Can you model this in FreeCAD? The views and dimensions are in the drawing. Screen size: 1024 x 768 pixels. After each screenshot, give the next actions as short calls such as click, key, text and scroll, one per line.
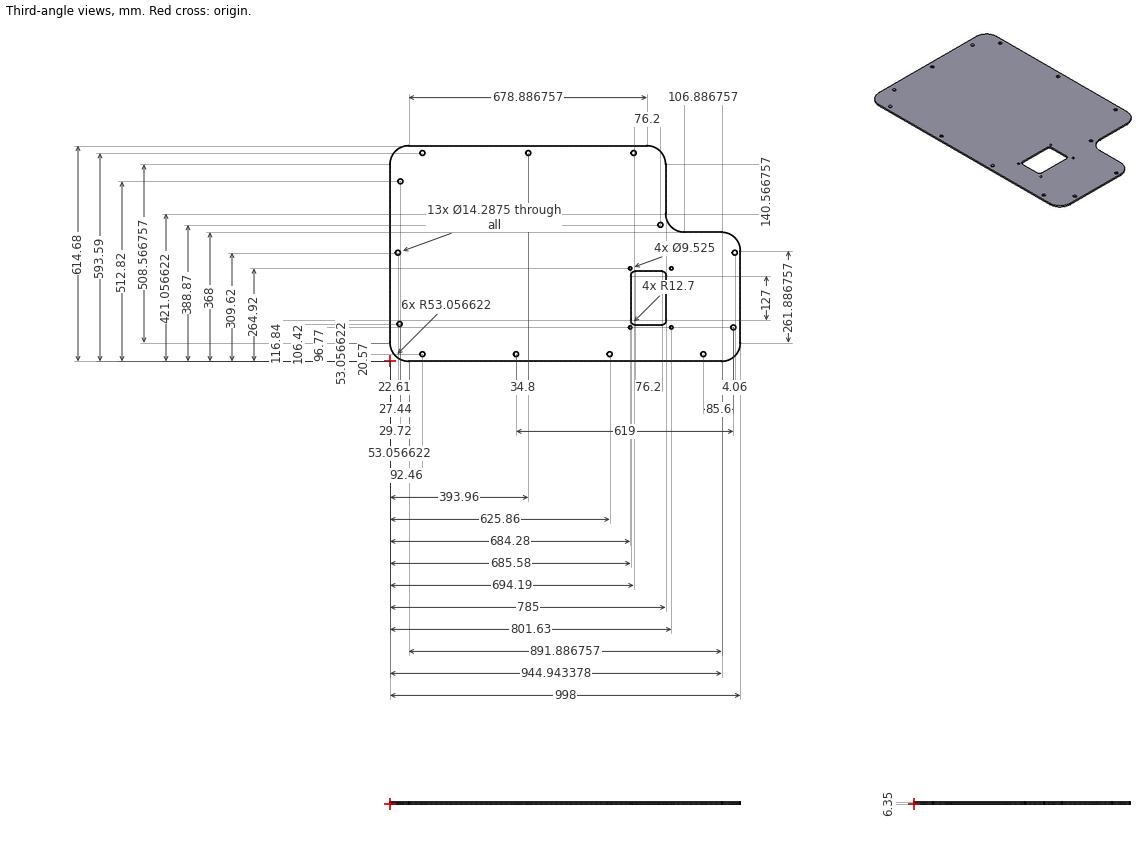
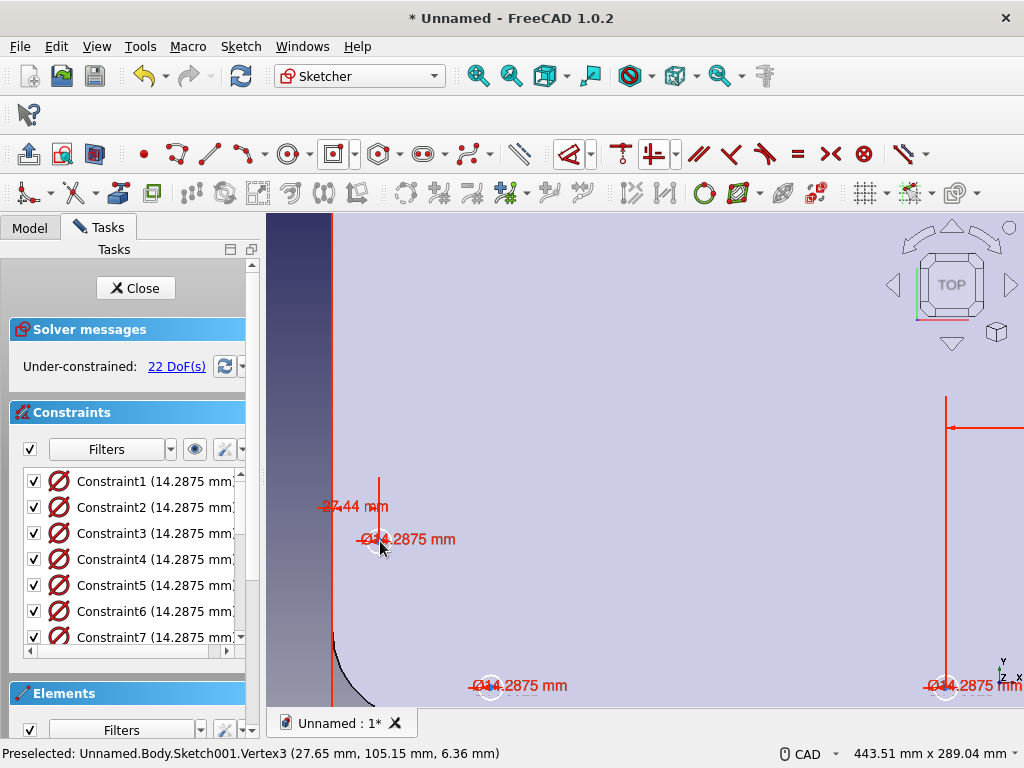
scroll(380, 543, down, 7)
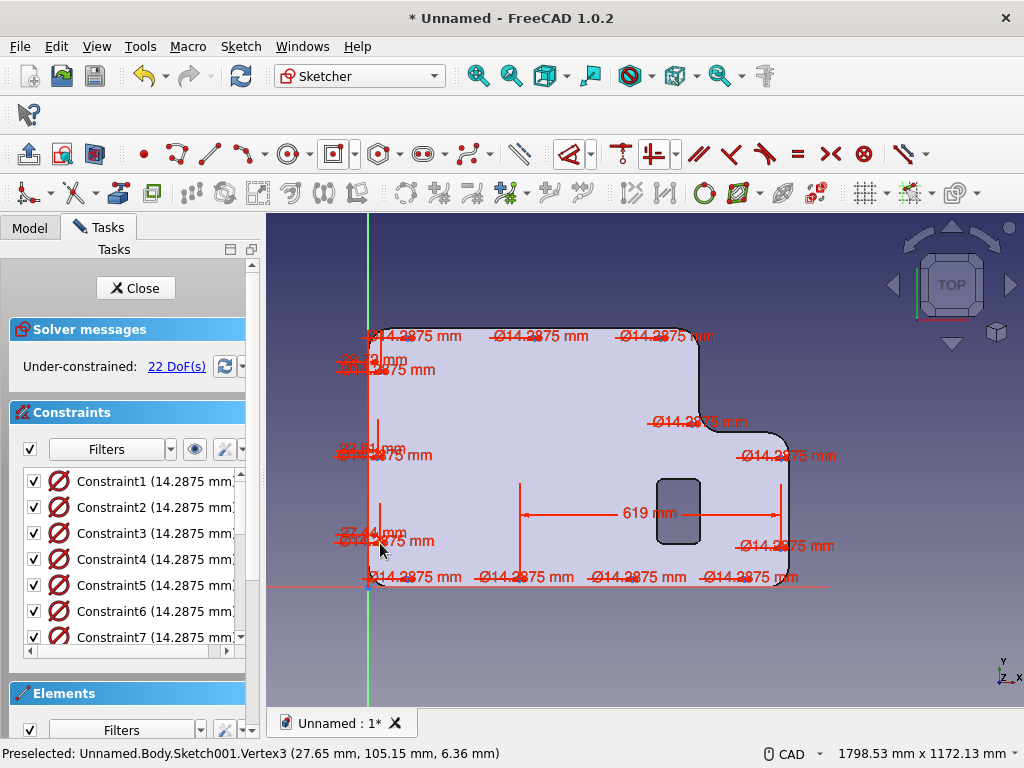
click(407, 579)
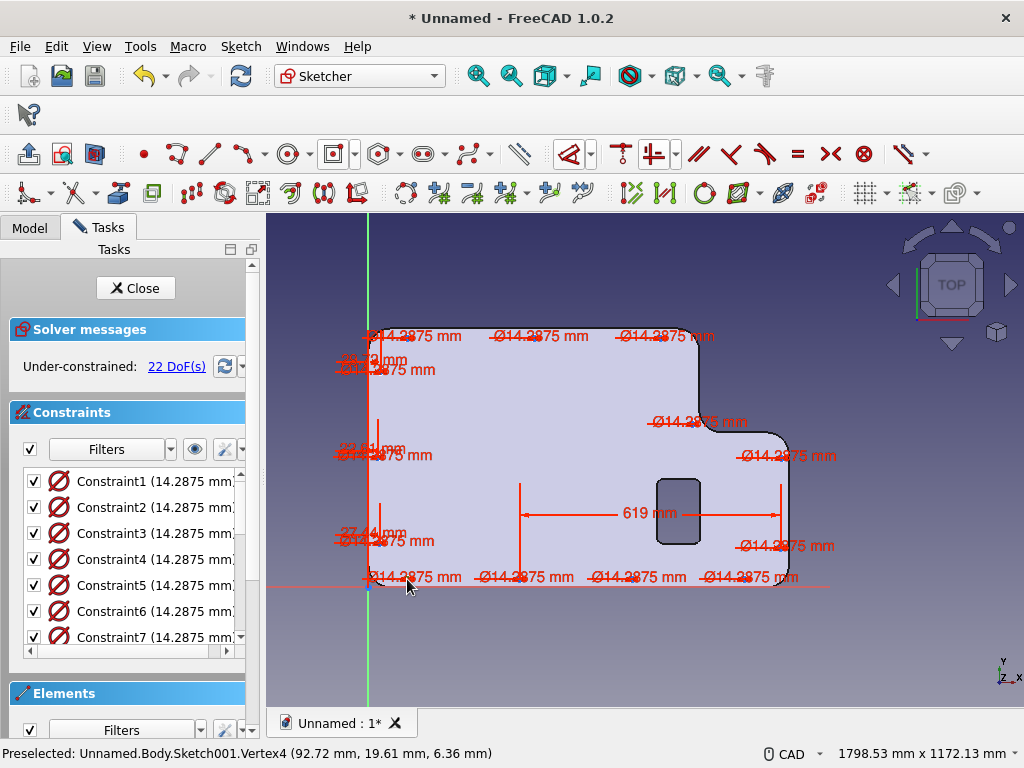
key(l)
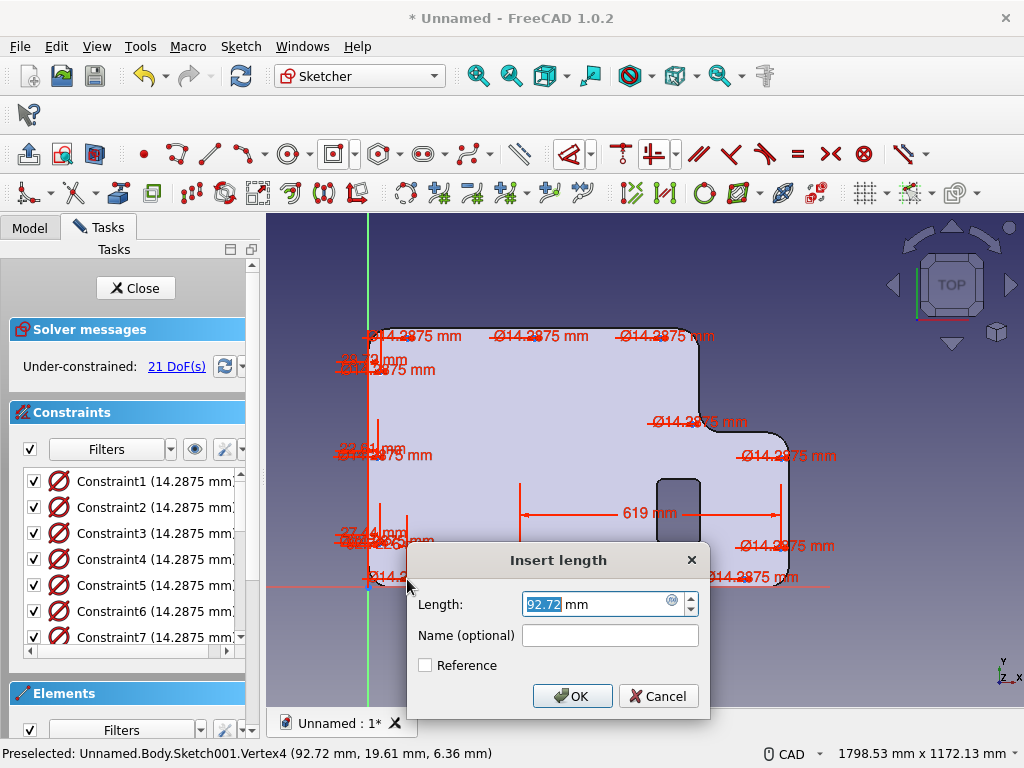
text(92.46)
key(Return)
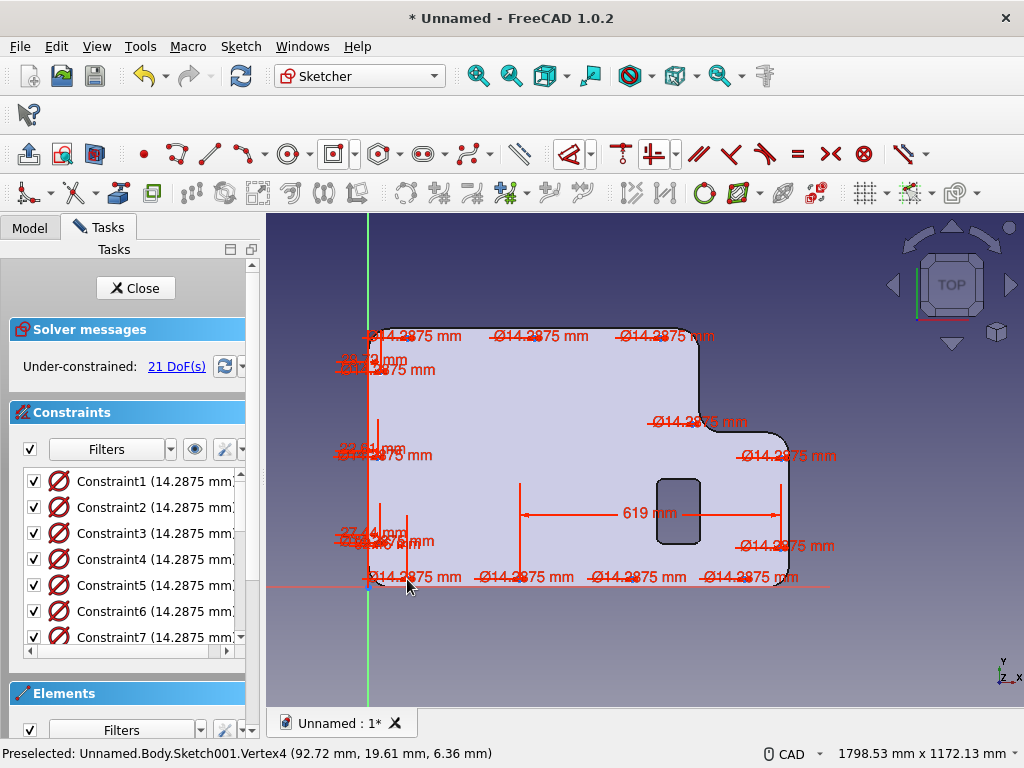
scroll(407, 579, up, 8)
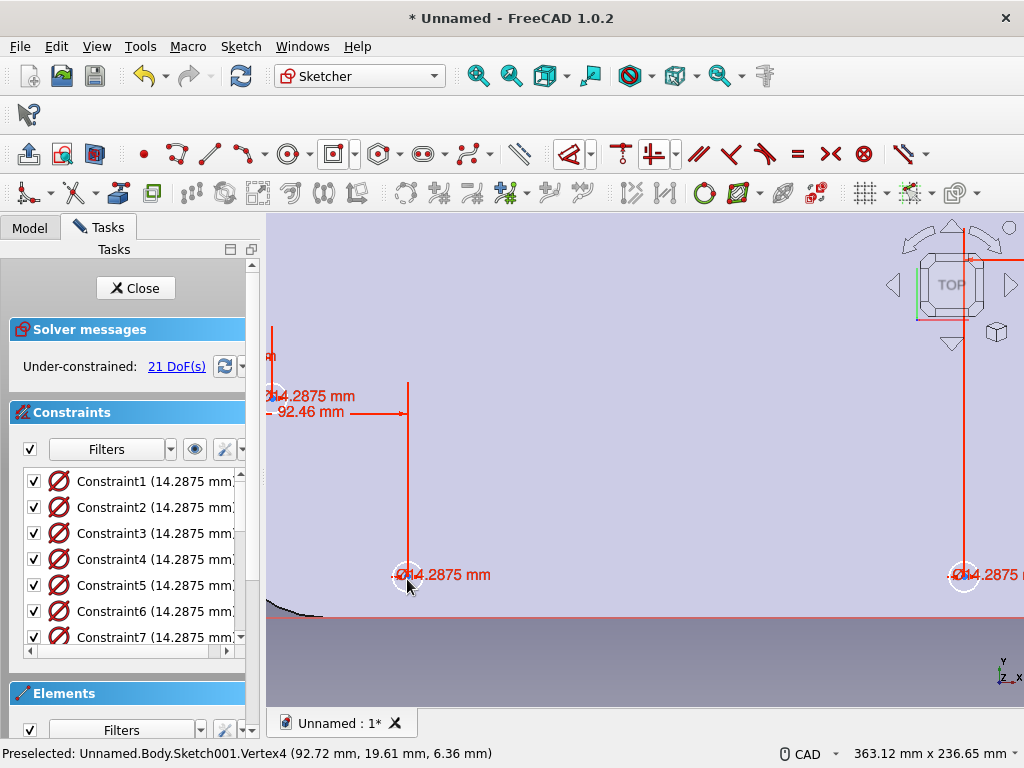
click(408, 577)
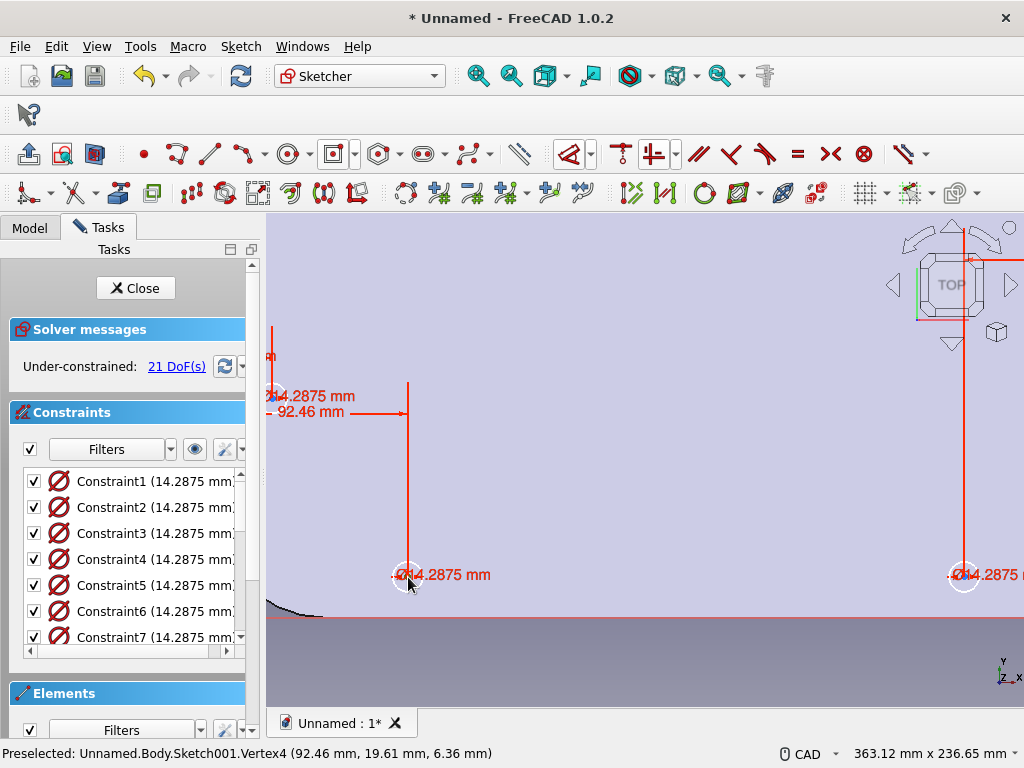
click(590, 154)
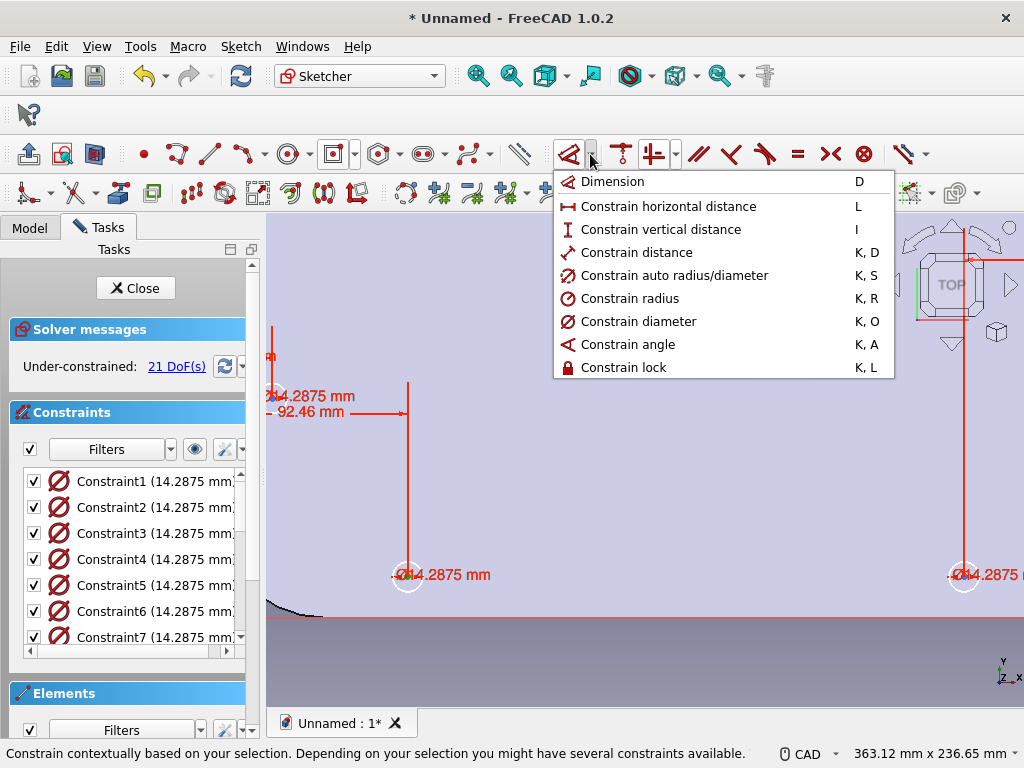
click(724, 230)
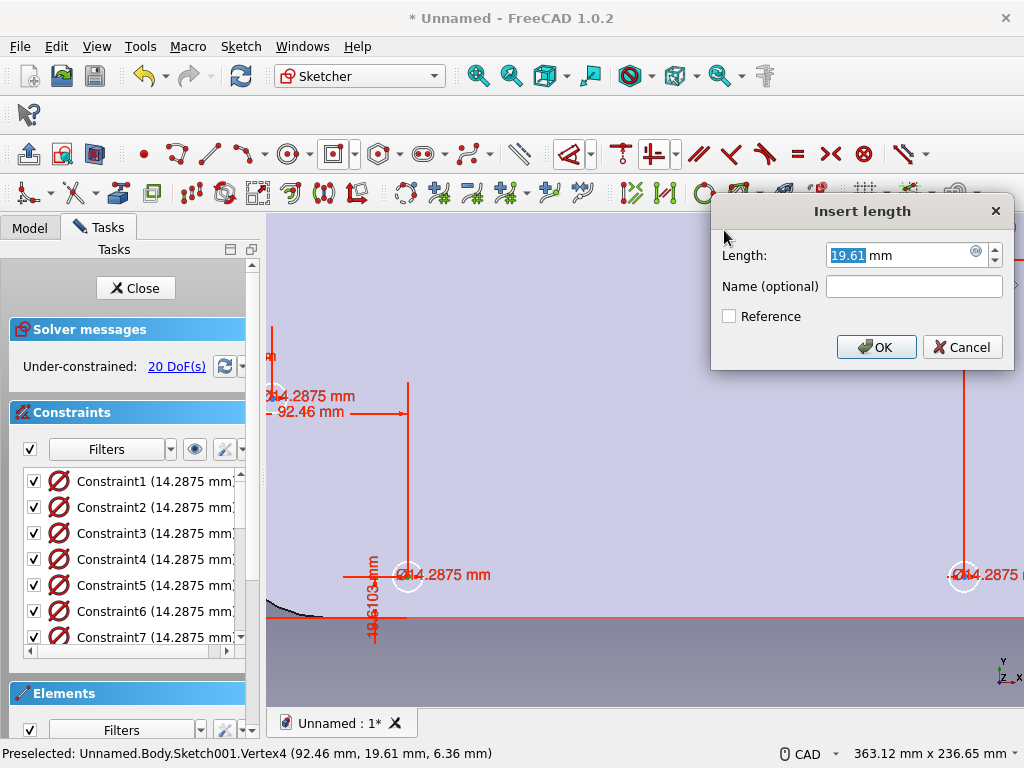
text(20.57)
key(Return)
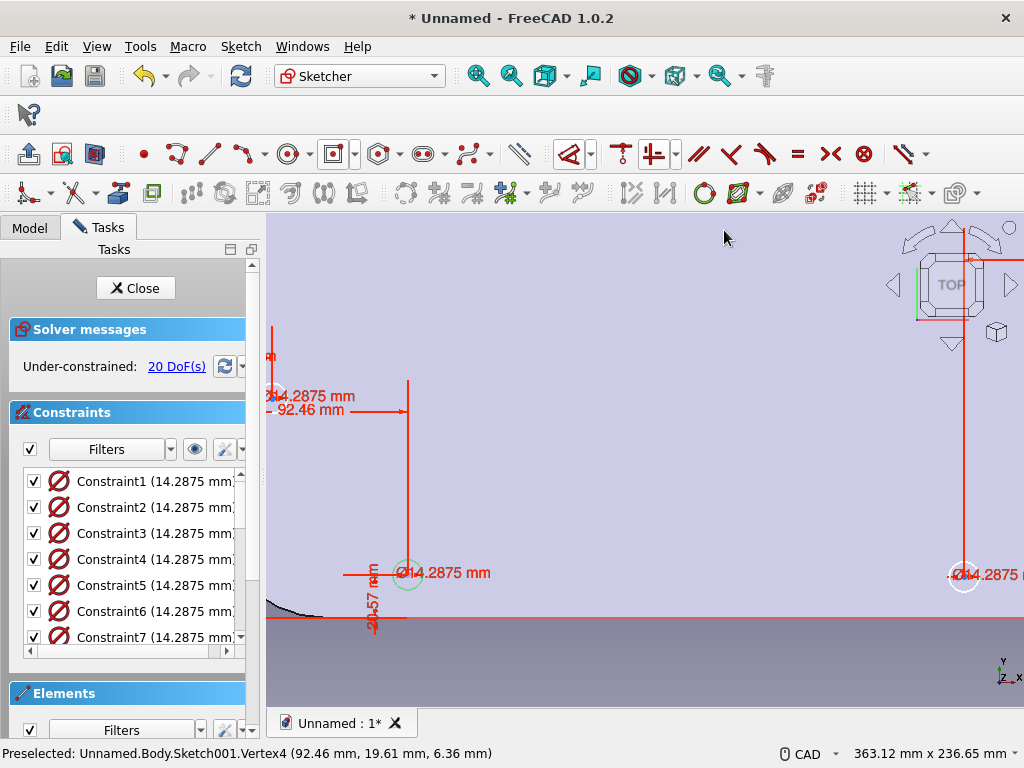
scroll(407, 579, down, 8)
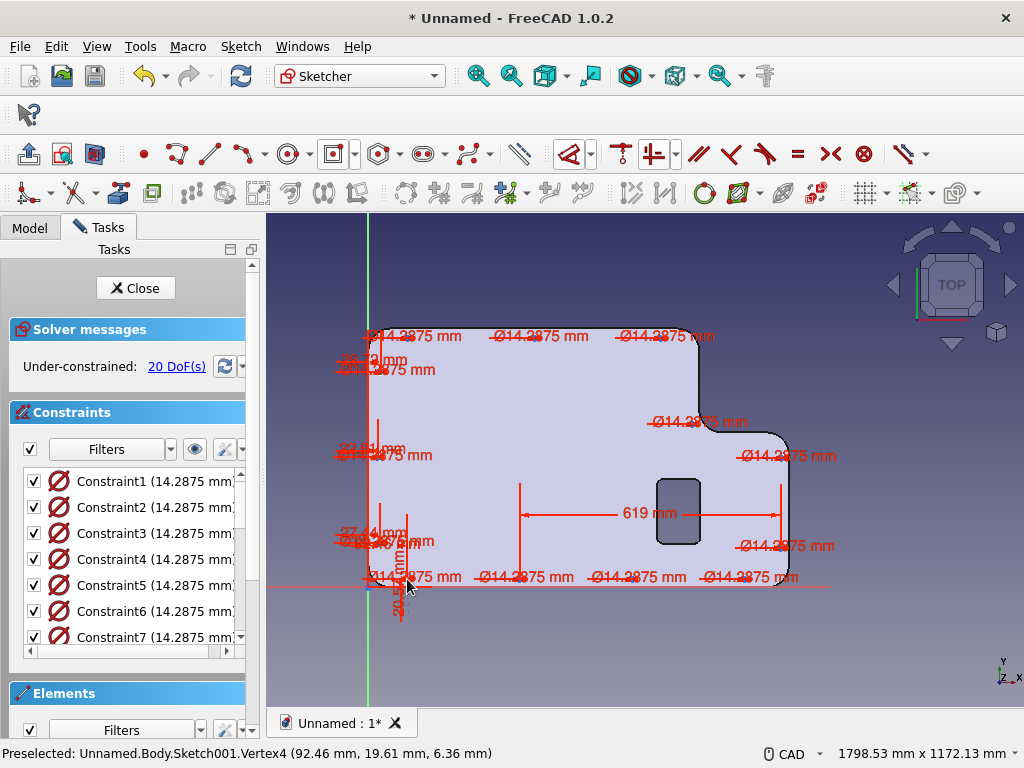
click(407, 338)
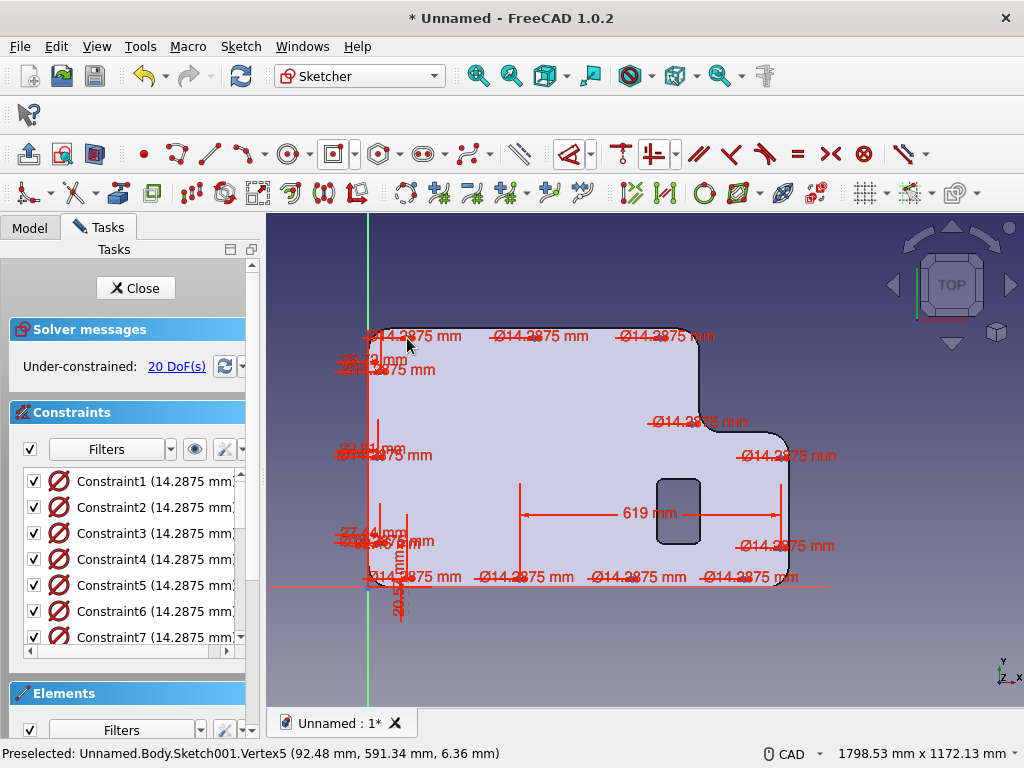
click(590, 154)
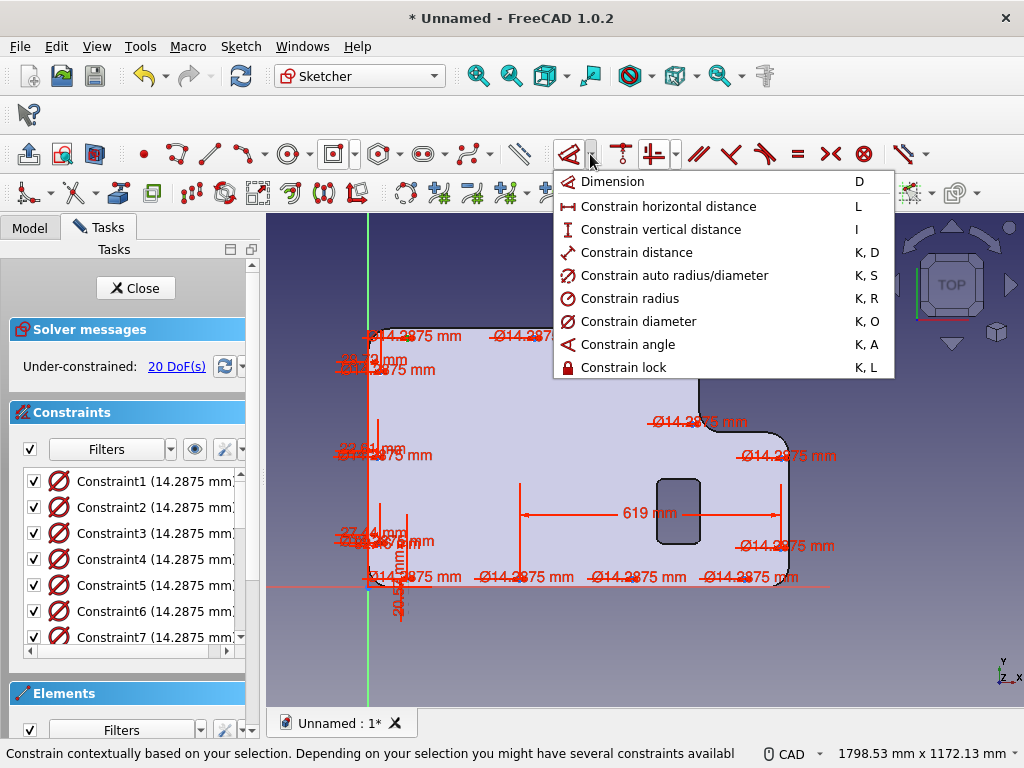
click(724, 206)